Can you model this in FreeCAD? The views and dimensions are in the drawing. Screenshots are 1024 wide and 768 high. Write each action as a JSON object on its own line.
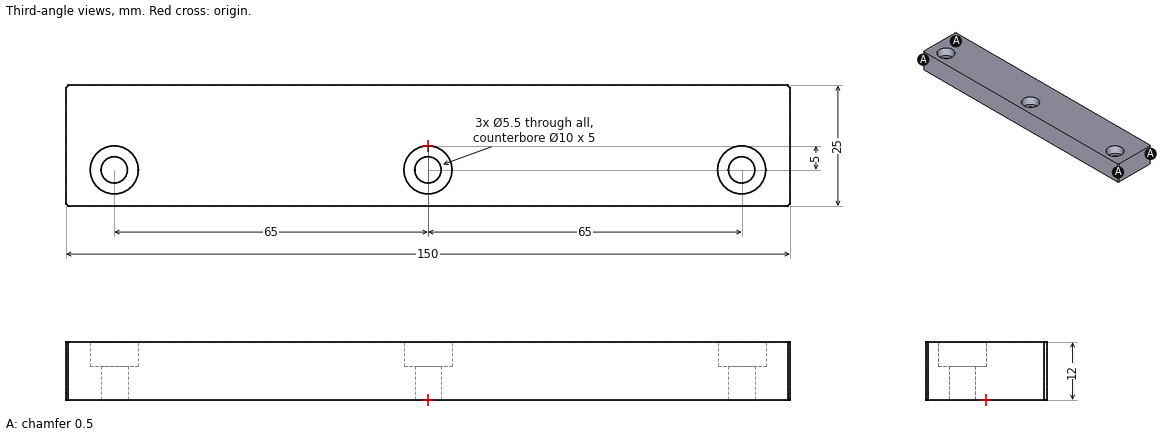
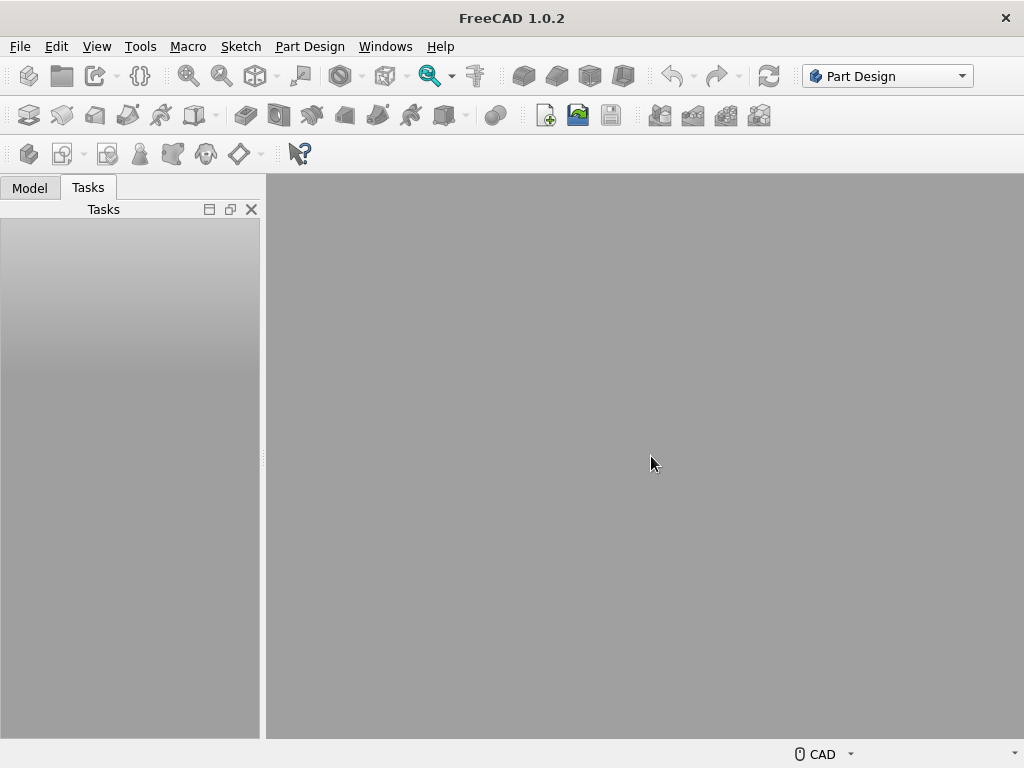
{"action": "left_click", "coordinate": [545, 116]}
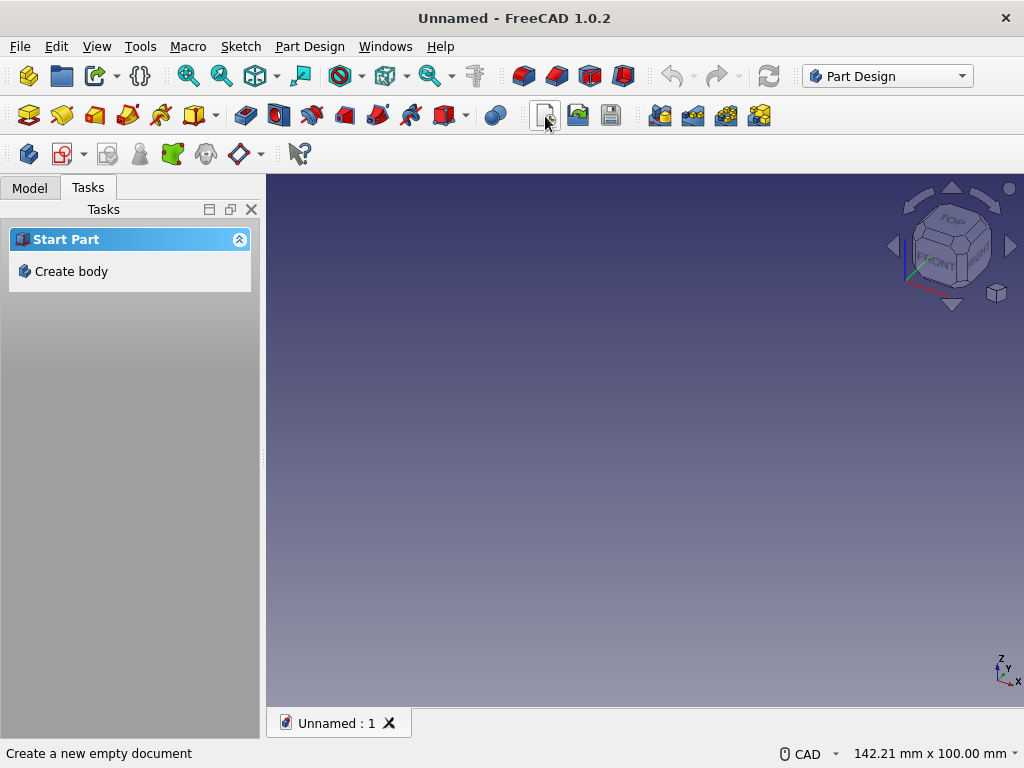
{"action": "left_click", "coordinate": [62, 154]}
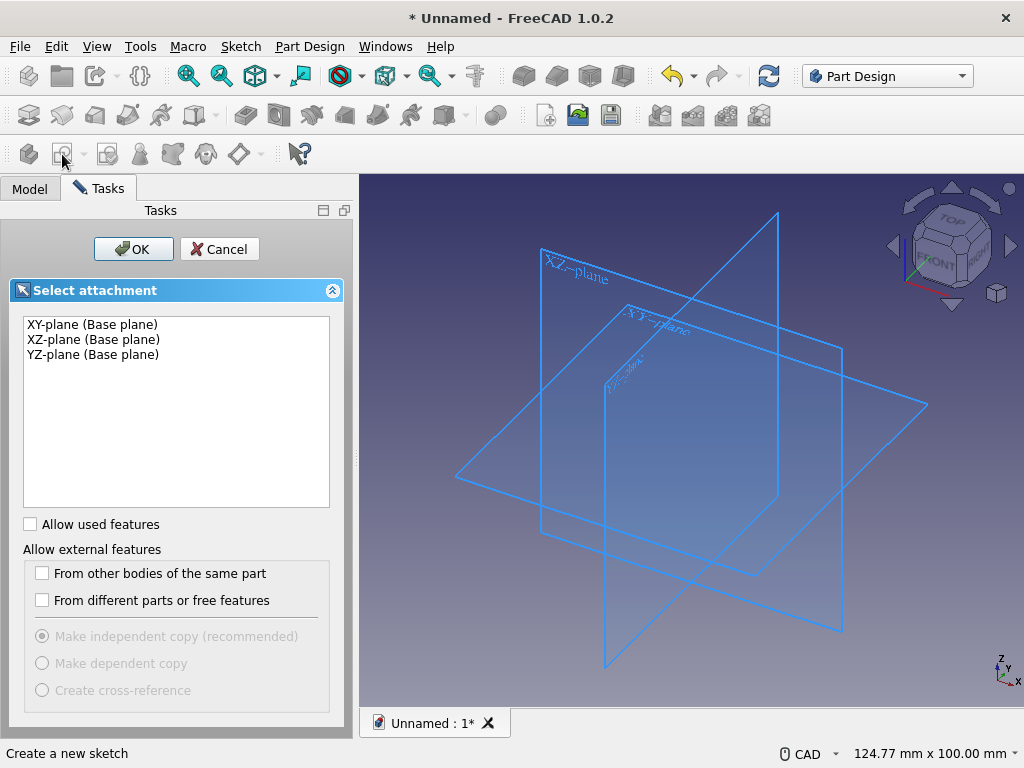
{"action": "left_click", "coordinate": [84, 324]}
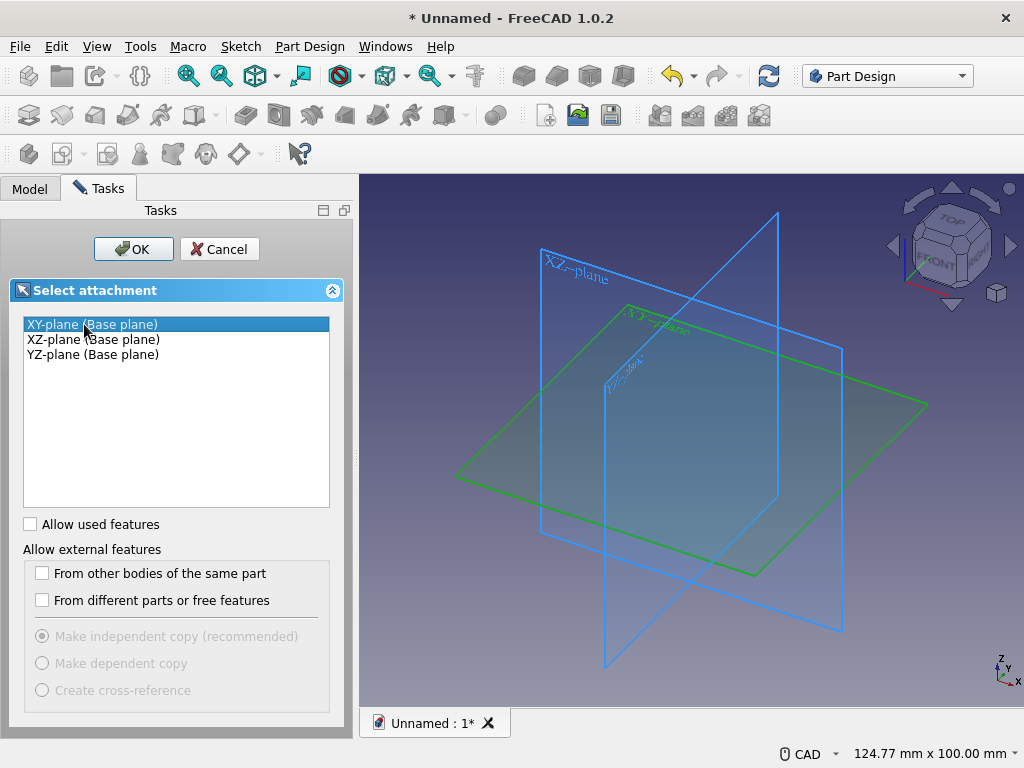
{"action": "left_click", "coordinate": [134, 249]}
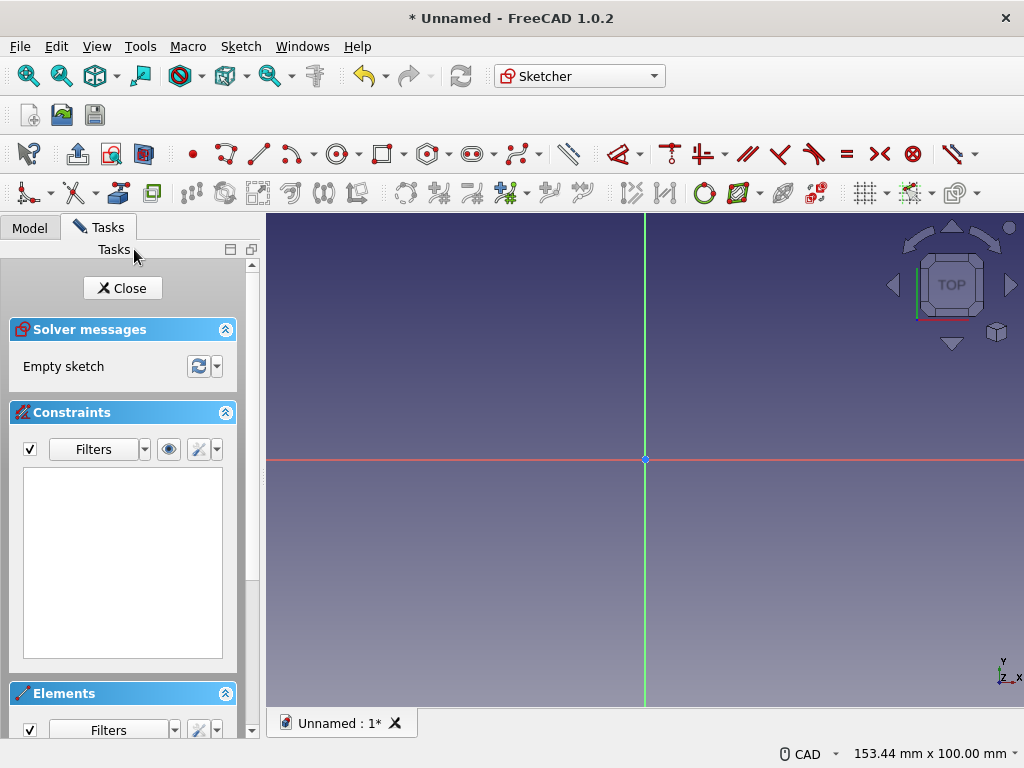
{"action": "scroll", "coordinate": [493, 460], "scroll_direction": "down", "scroll_amount": 3}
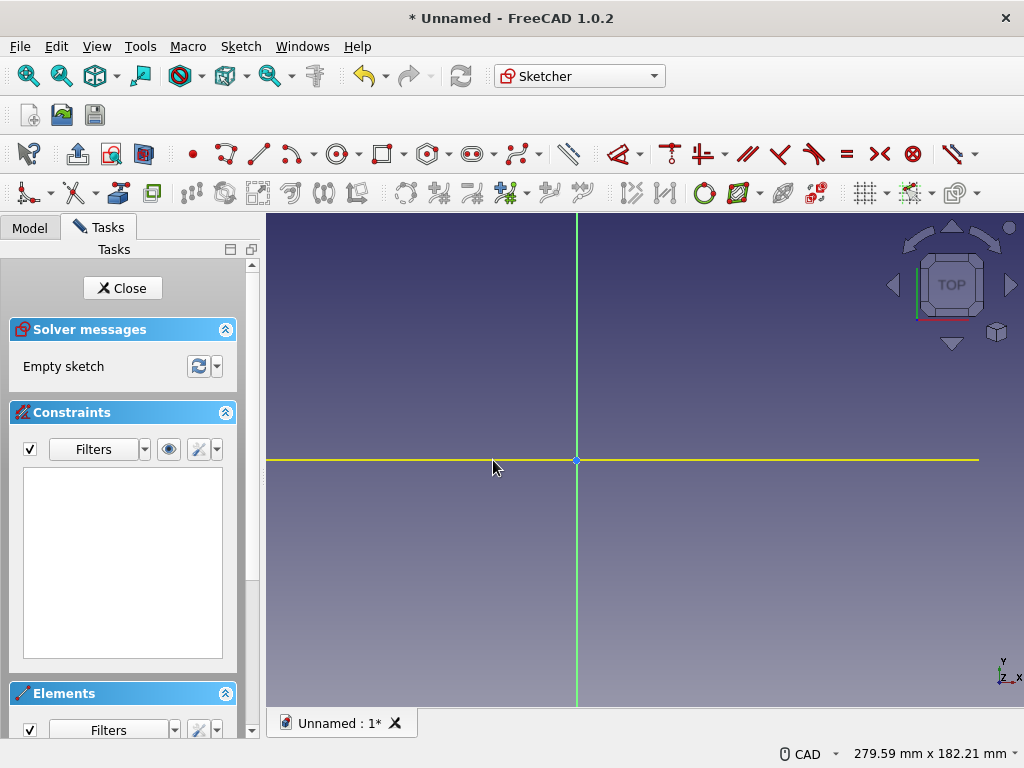
{"action": "key", "text": "g v"}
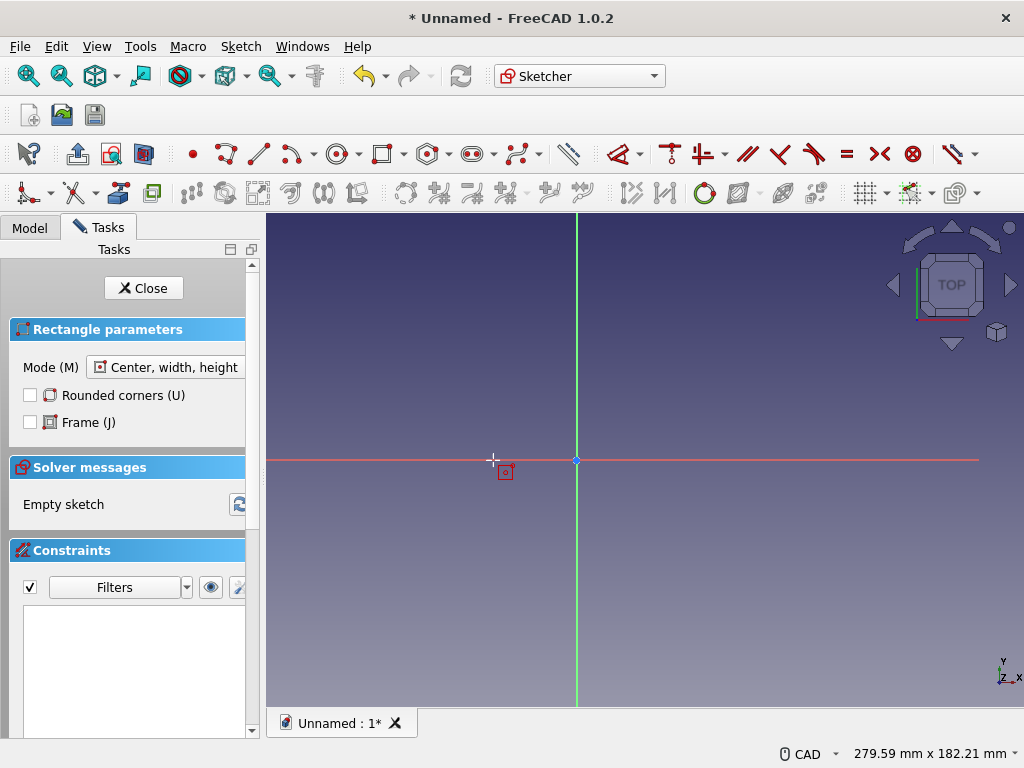
{"action": "left_click", "coordinate": [577, 460]}
{"action": "left_click", "coordinate": [780, 426]}
{"action": "key", "text": "Escape"}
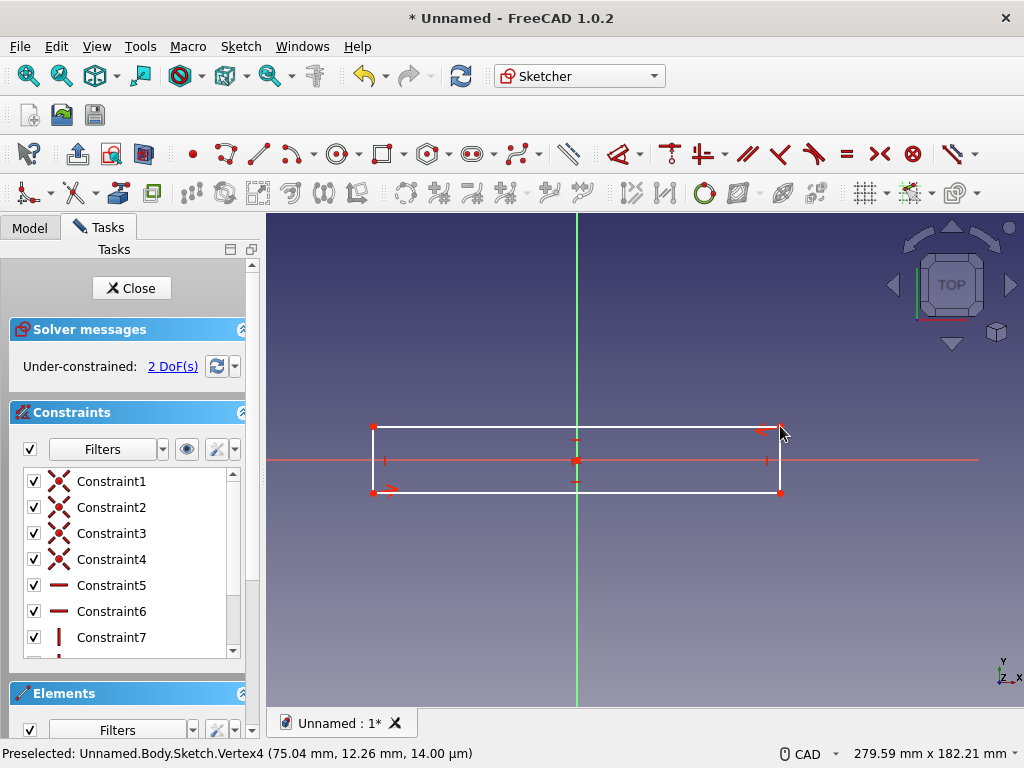
{"action": "left_click", "coordinate": [618, 154]}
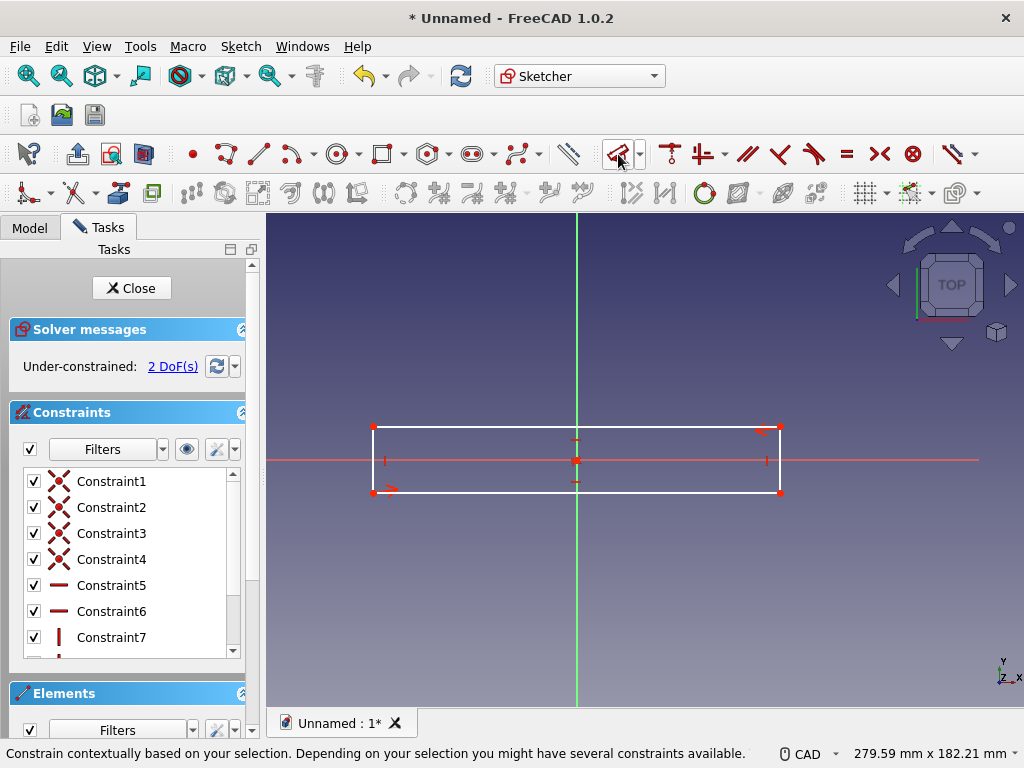
{"action": "left_click", "coordinate": [780, 474]}
{"action": "left_click", "coordinate": [814, 445]}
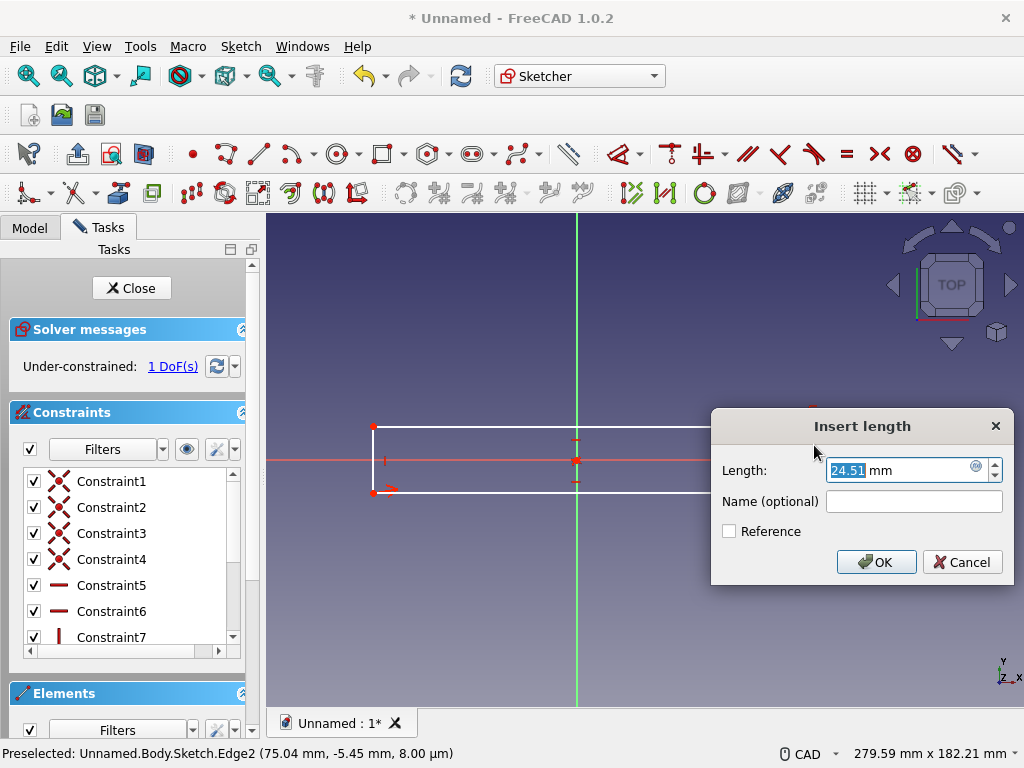
{"action": "type", "text": "25"}
{"action": "key", "text": "Return"}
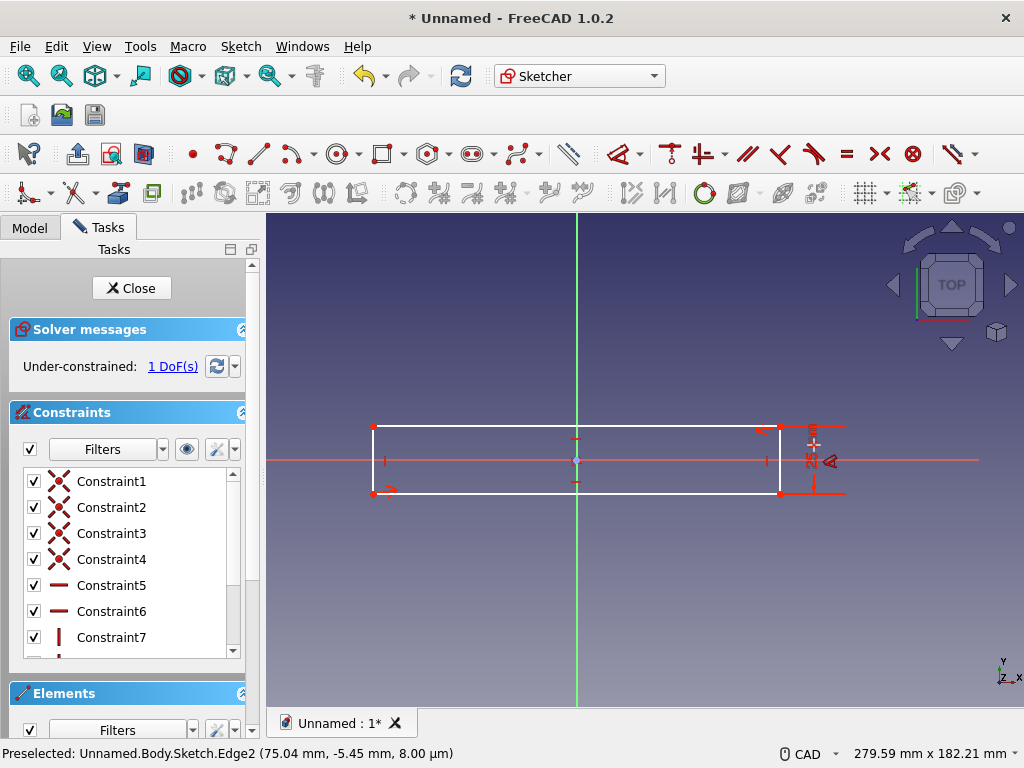
{"action": "left_click", "coordinate": [495, 494]}
{"action": "left_click", "coordinate": [483, 528]}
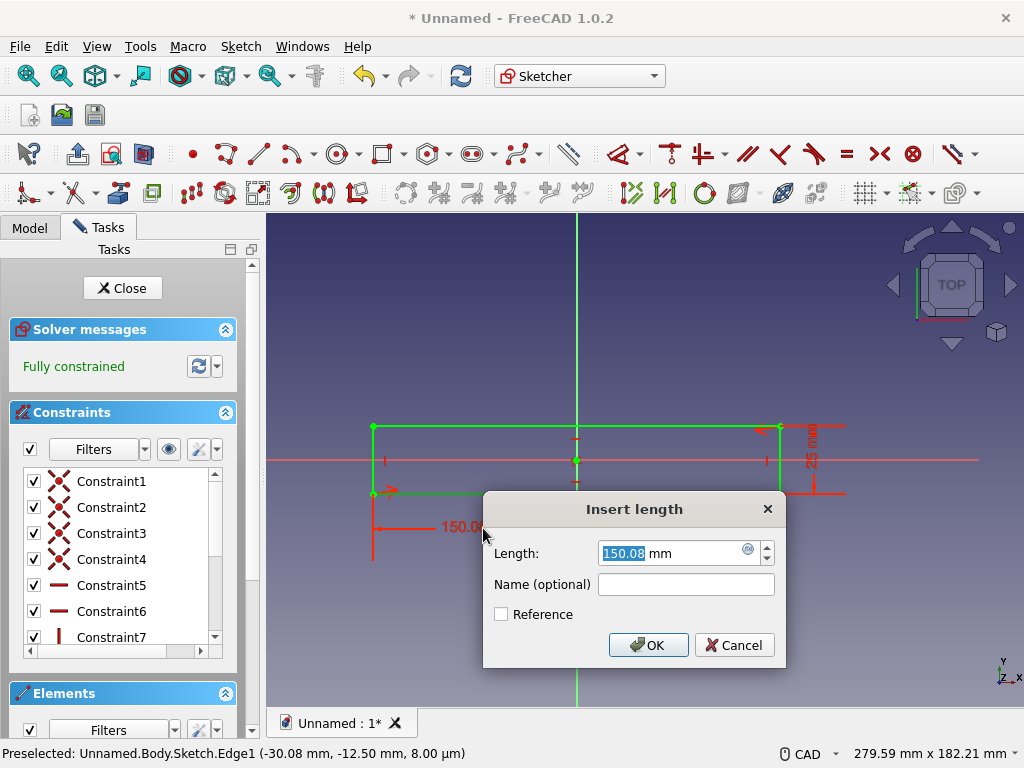
{"action": "type", "text": "150"}
{"action": "key", "text": "Return"}
{"action": "key", "text": "Escape"}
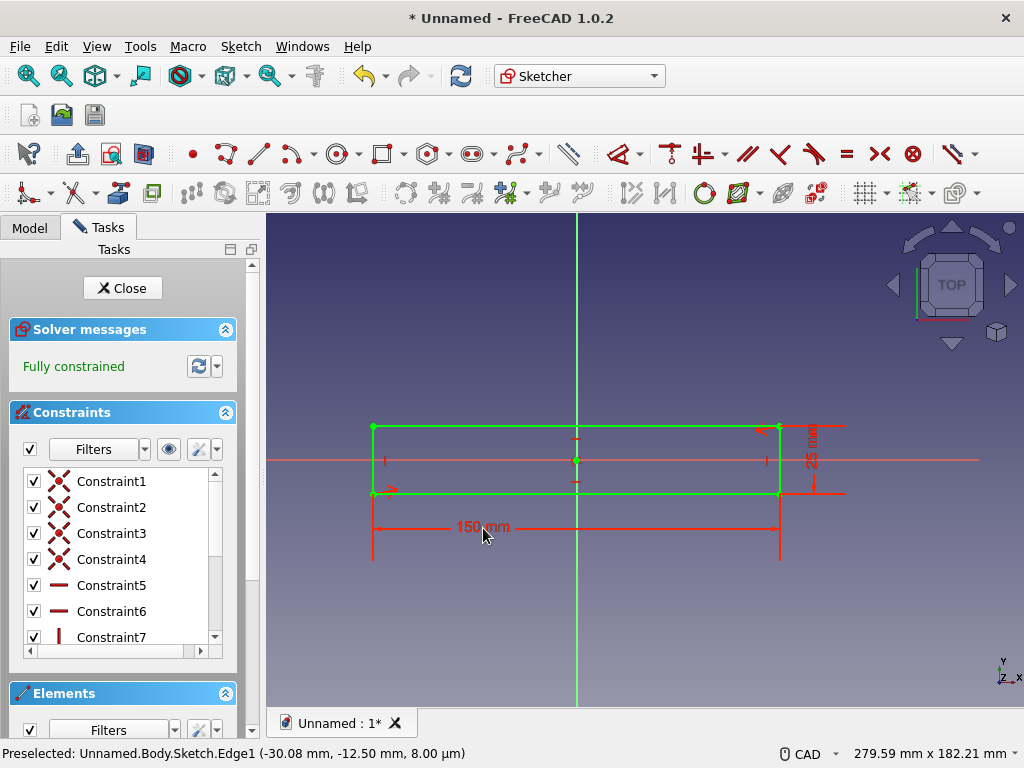
{"action": "left_click", "coordinate": [123, 288]}